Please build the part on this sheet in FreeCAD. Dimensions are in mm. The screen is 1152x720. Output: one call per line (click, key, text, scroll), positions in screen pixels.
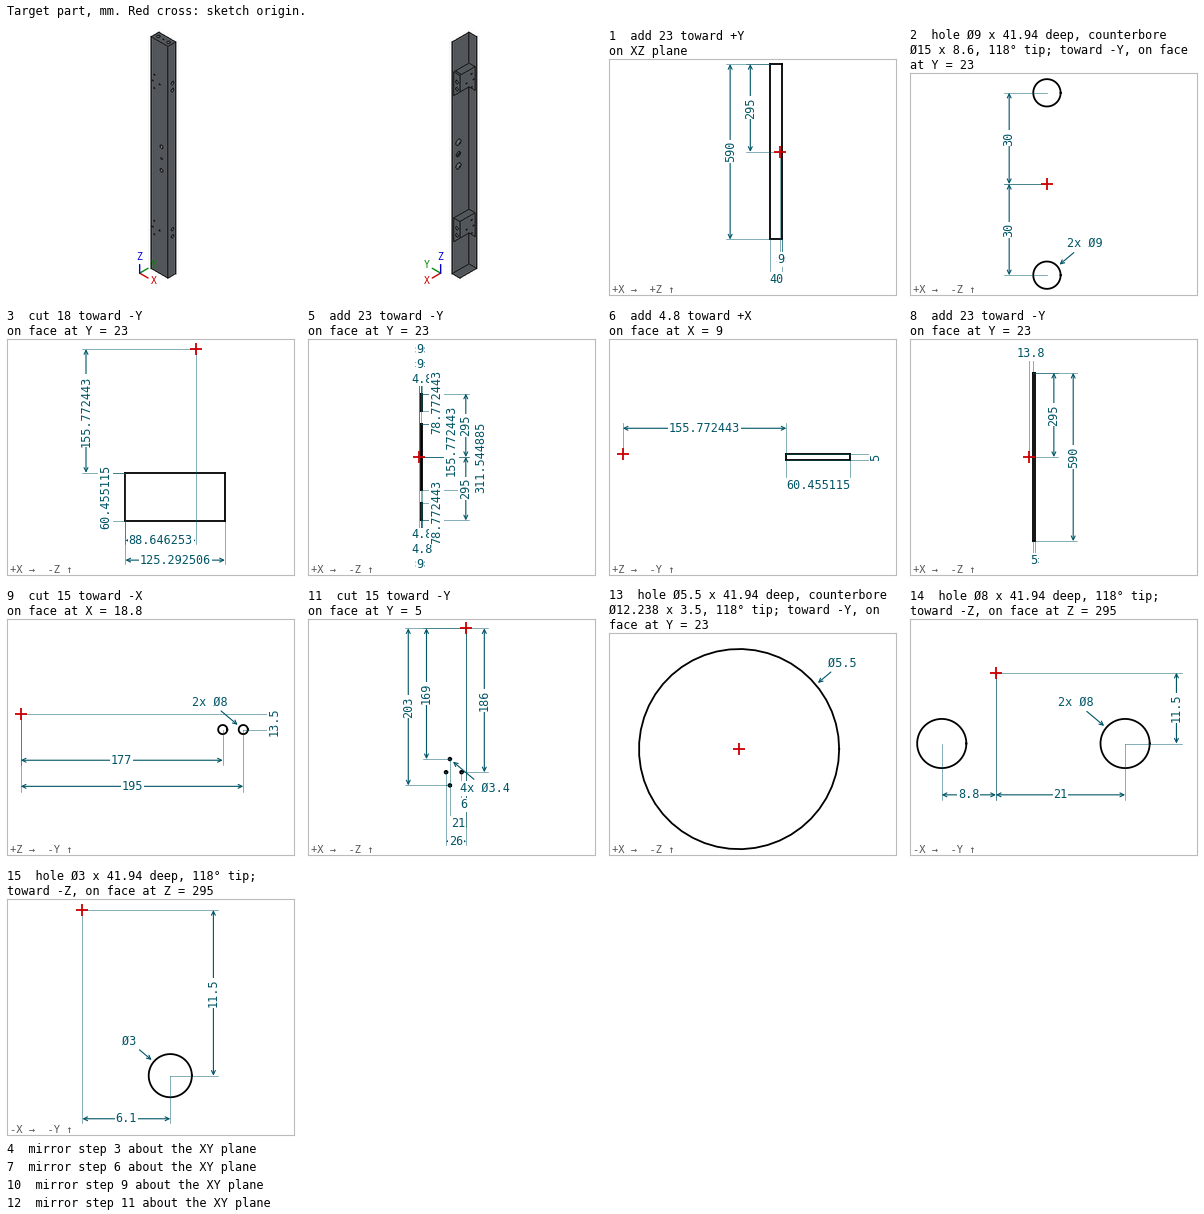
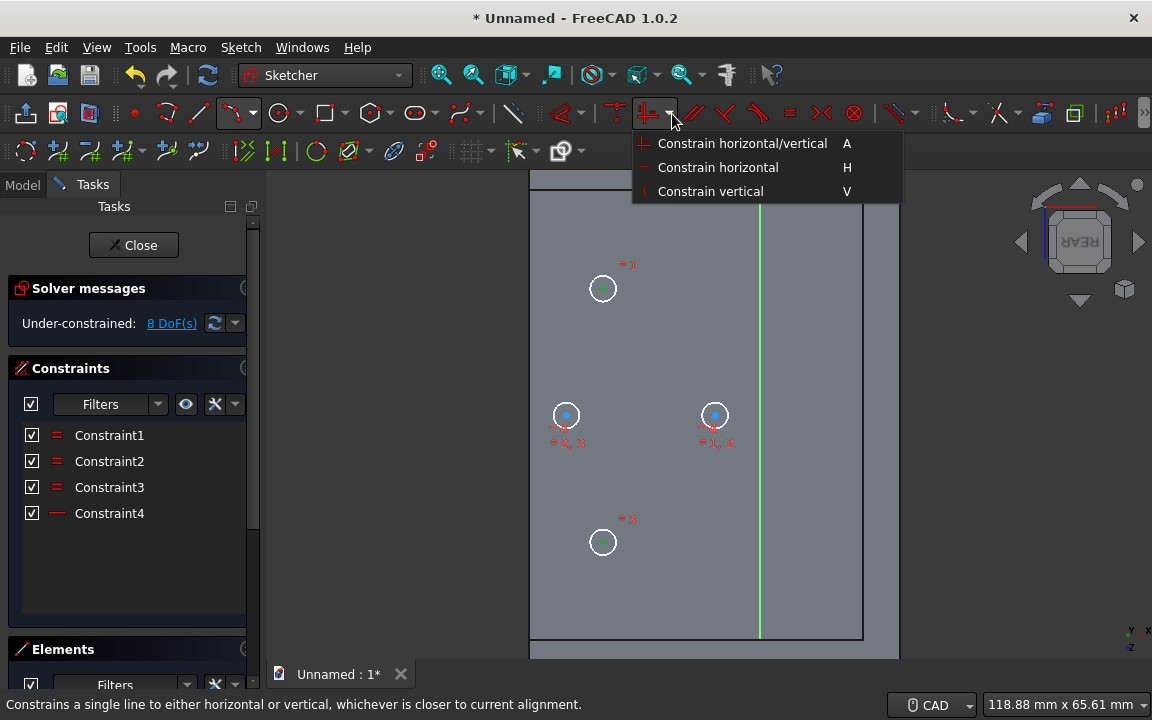
click(768, 191)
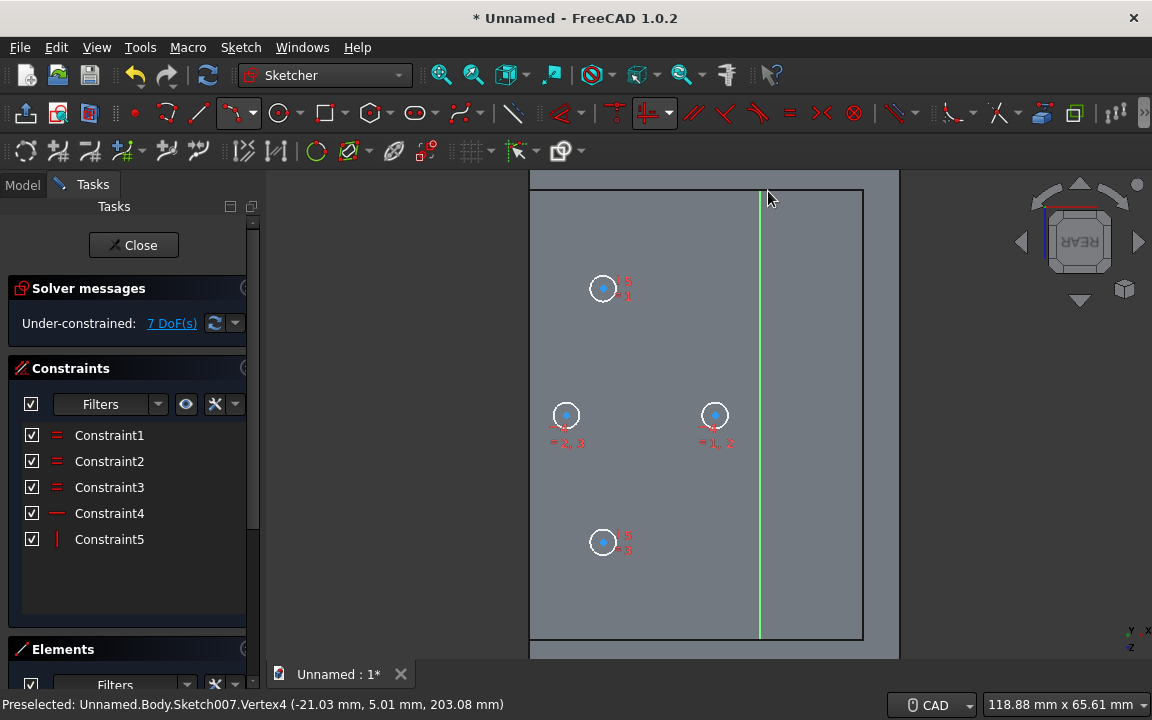
click(560, 114)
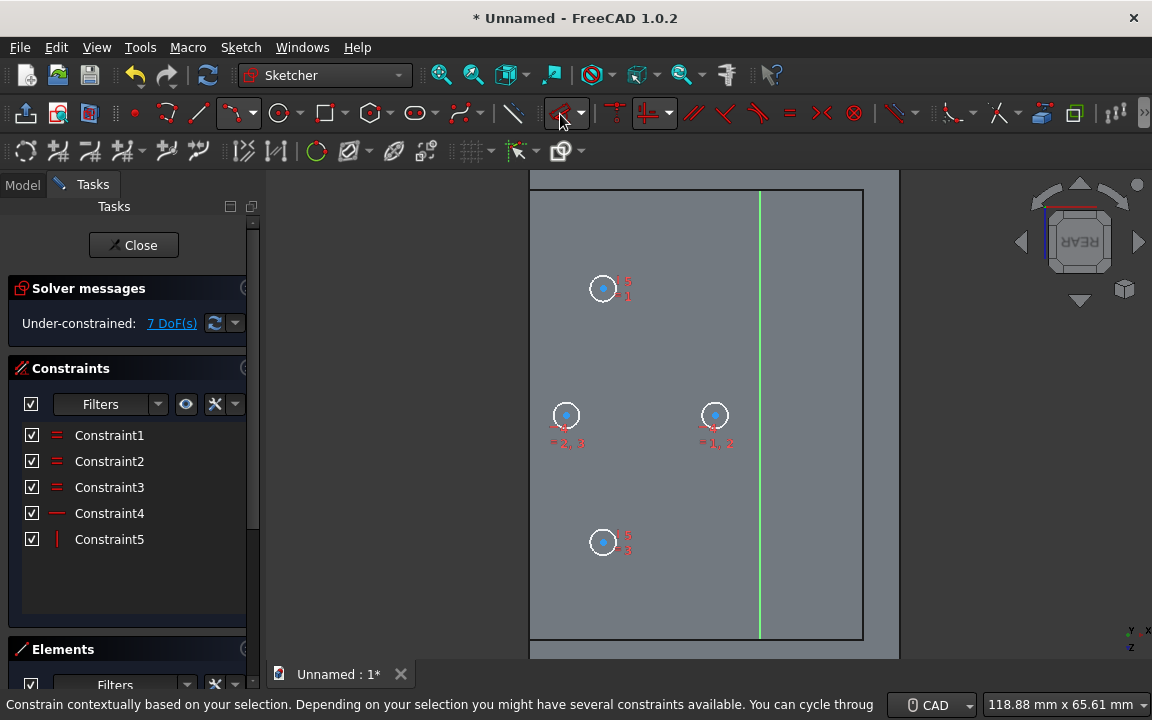
scroll(612, 280, up, 3)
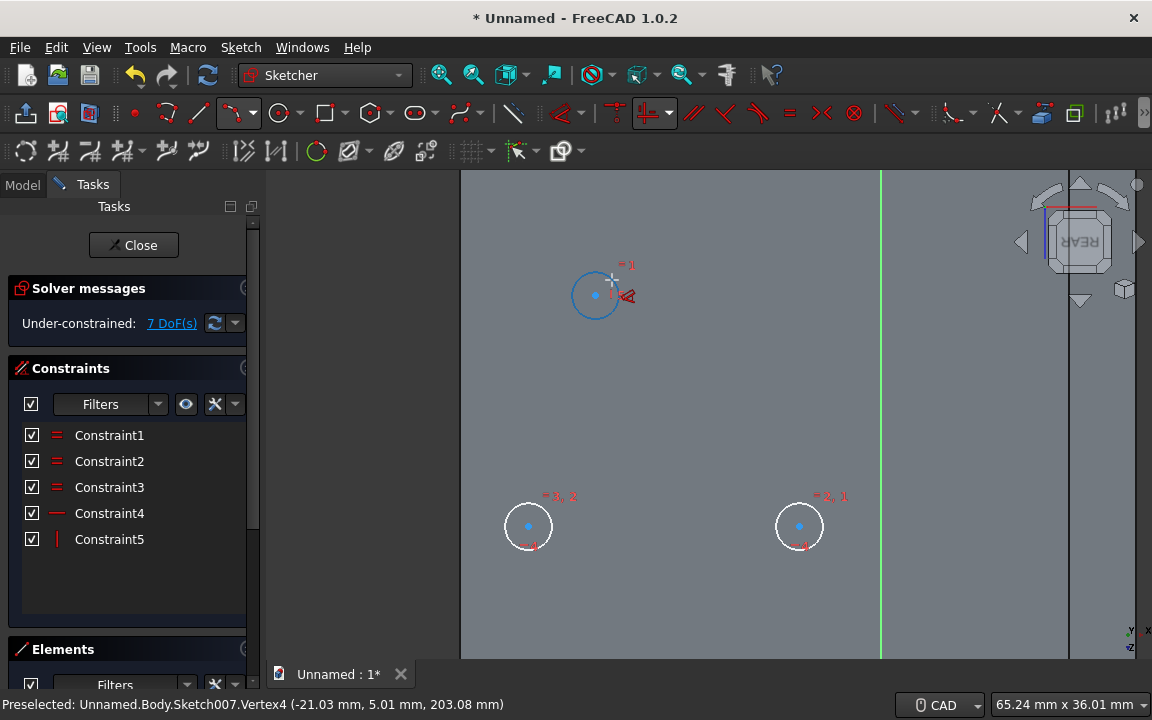
click(612, 279)
click(634, 256)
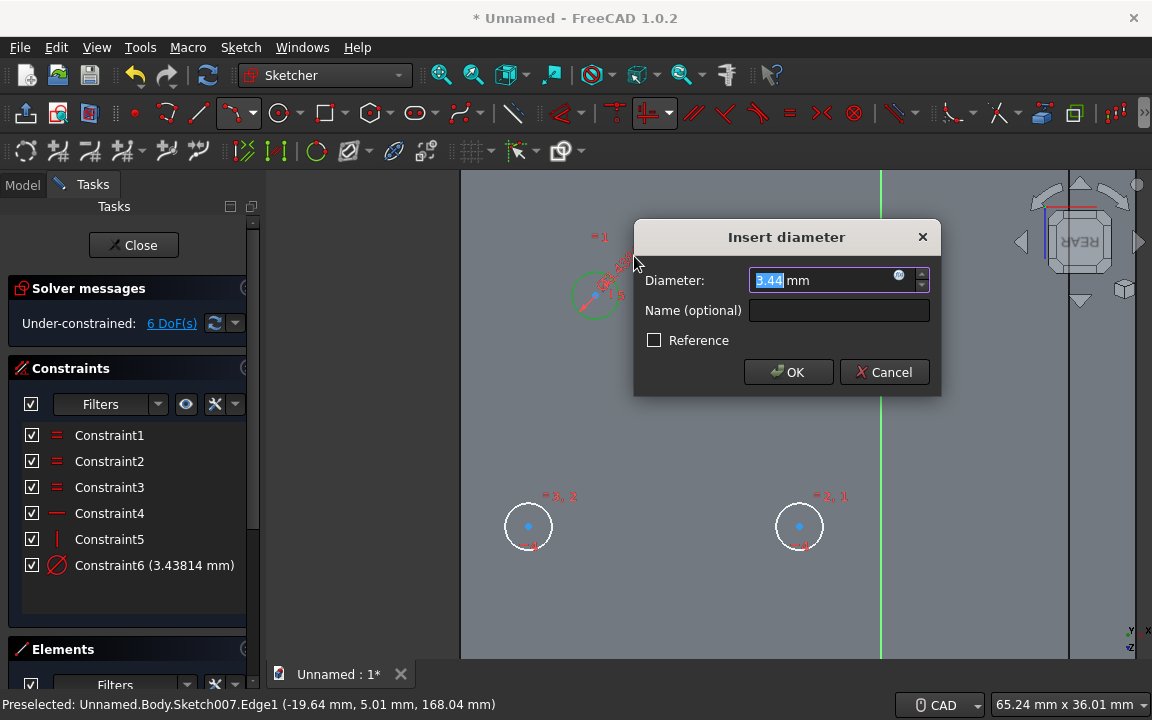
text(3.4)
key(Return)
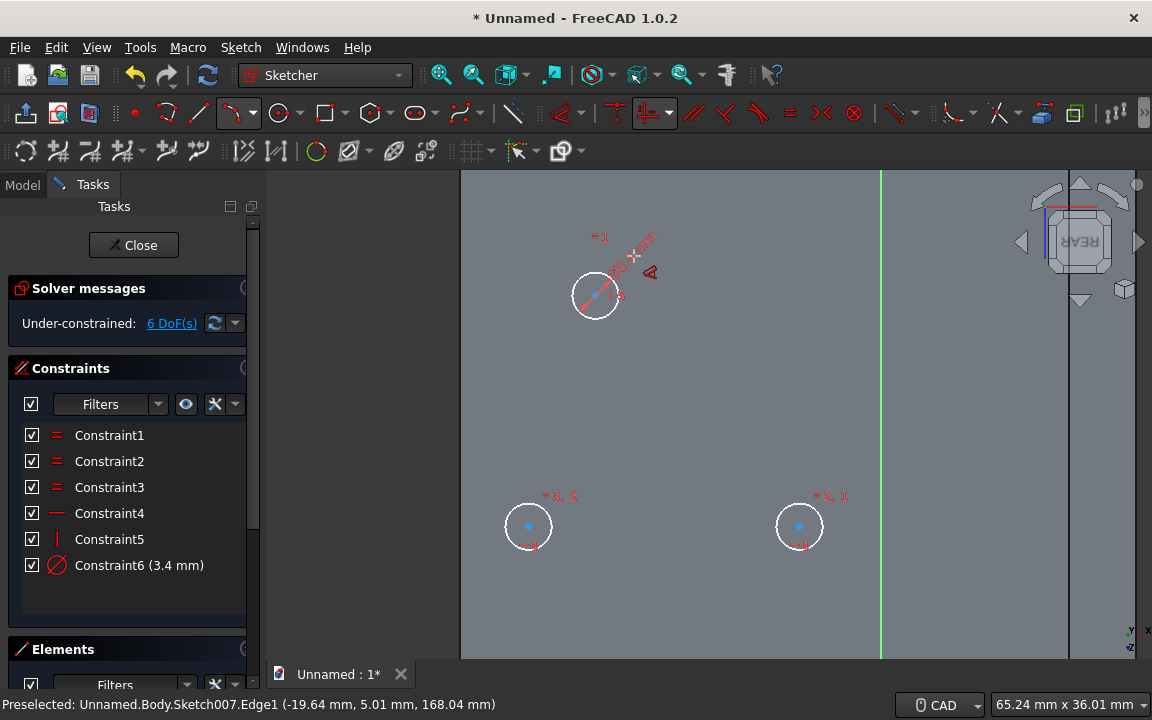
click(800, 527)
click(840, 561)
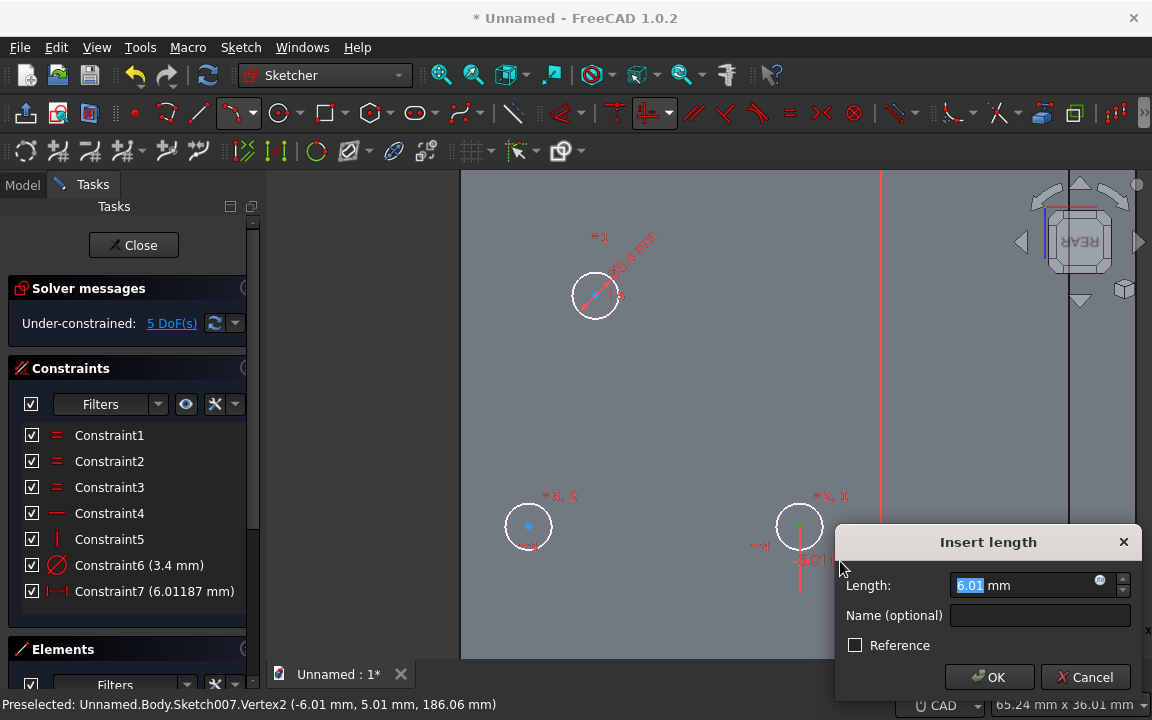
text(6)
key(Return)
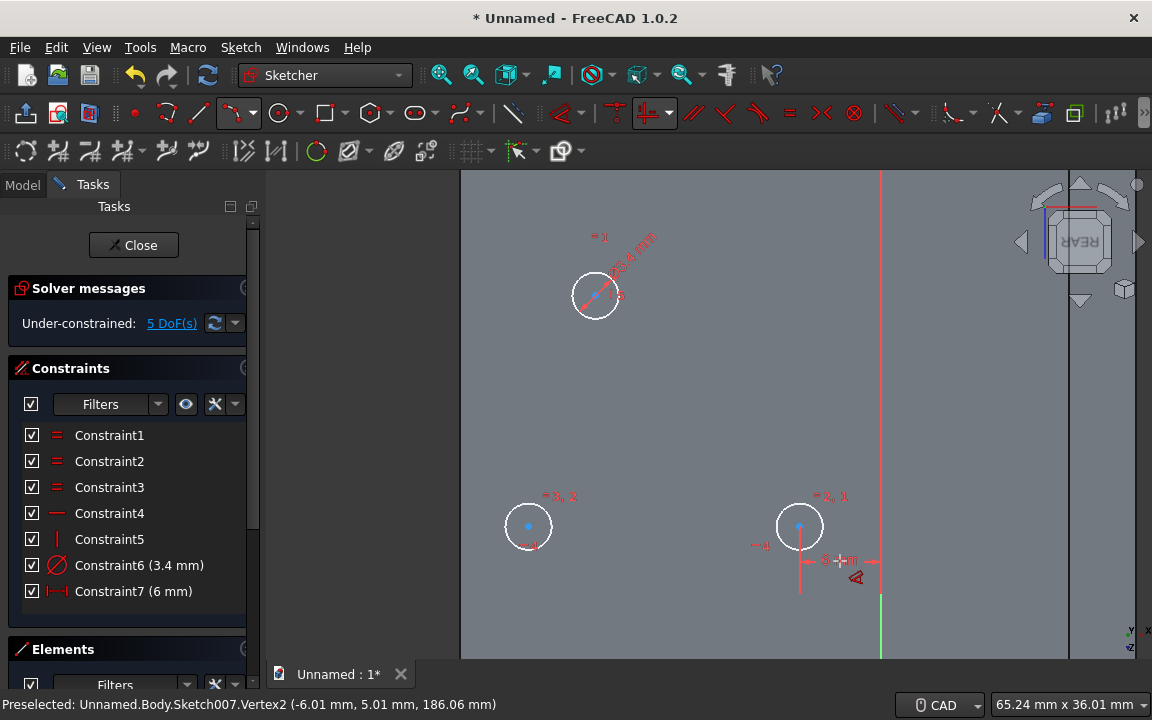
click(596, 296)
click(738, 330)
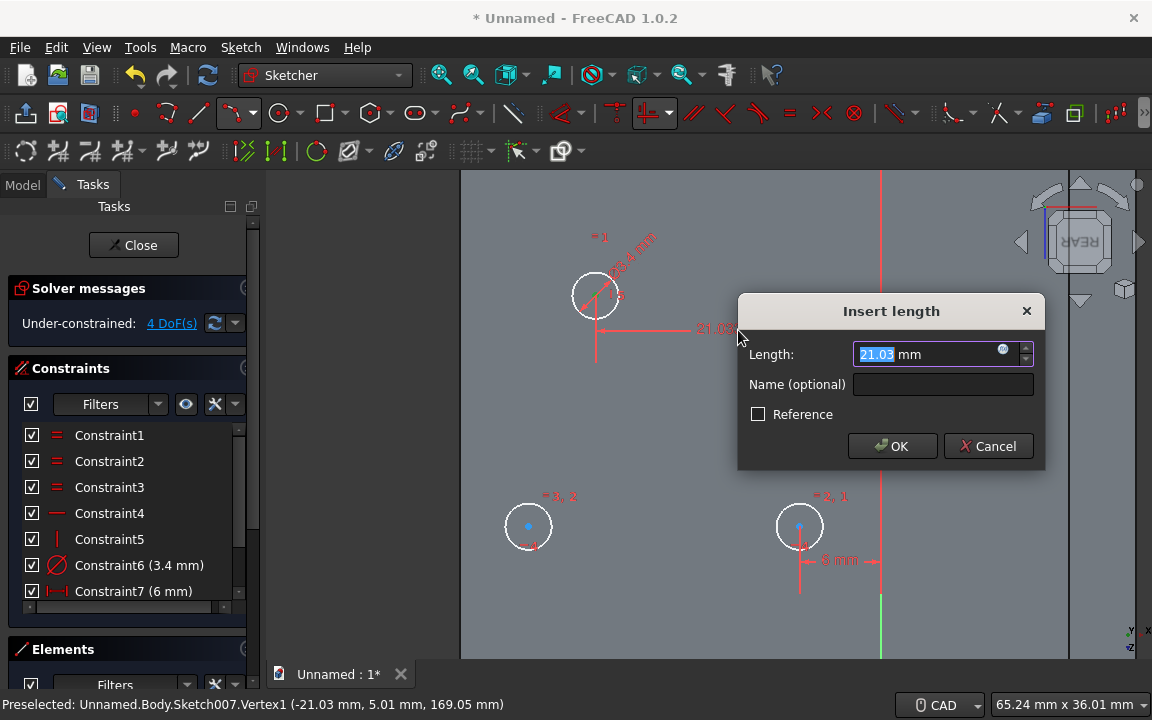
text(21)
key(Return)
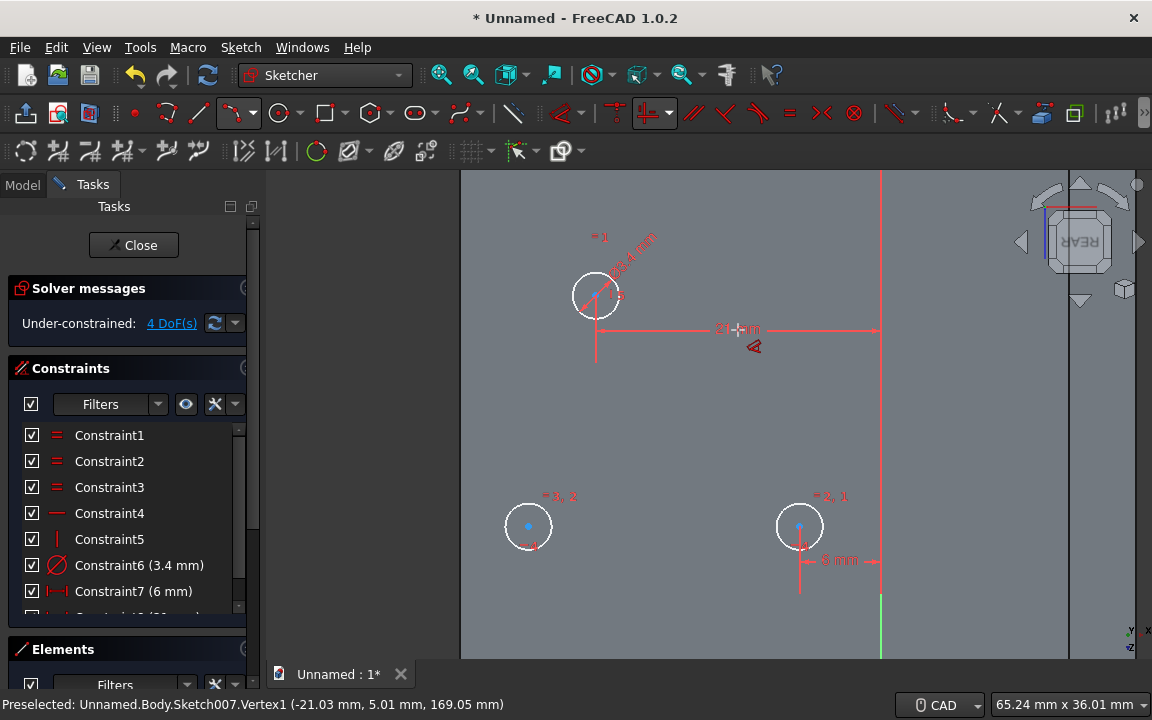
click(529, 527)
click(705, 561)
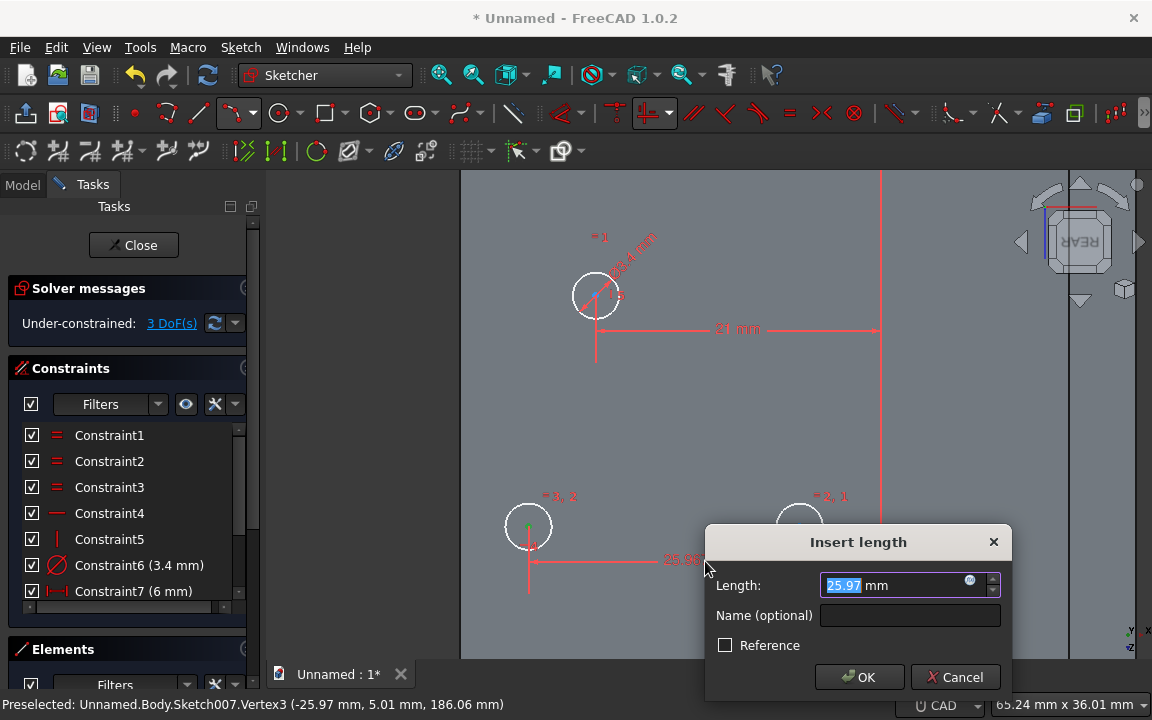
text(26)
key(Return)